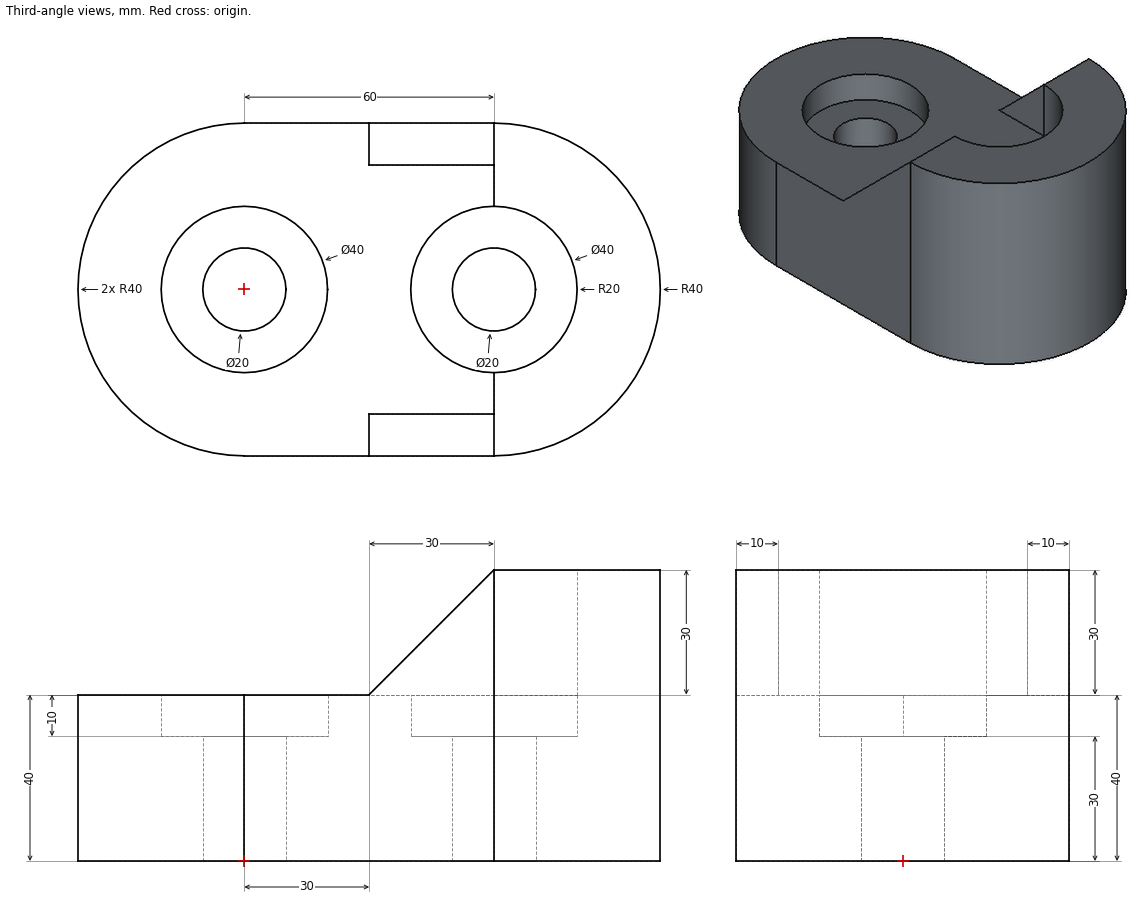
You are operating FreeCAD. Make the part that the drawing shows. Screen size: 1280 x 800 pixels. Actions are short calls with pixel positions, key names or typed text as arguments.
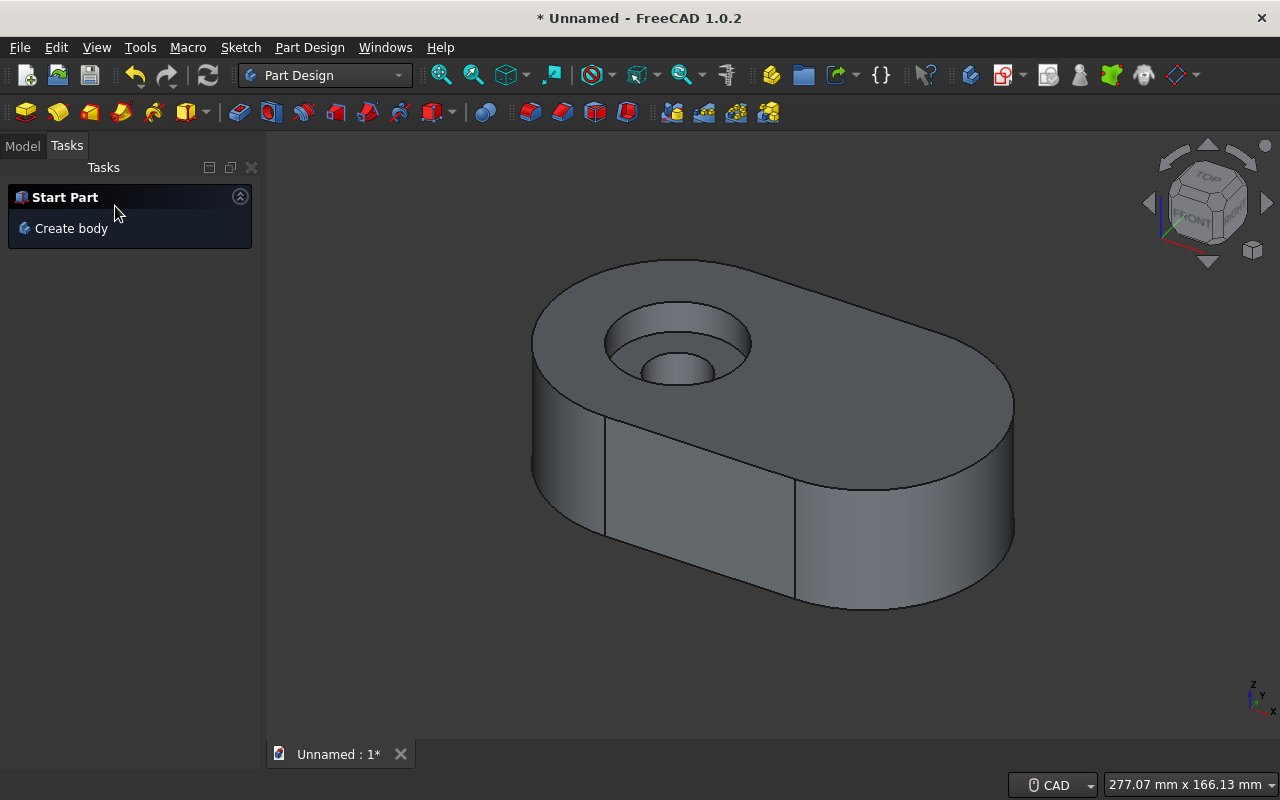
click(900, 416)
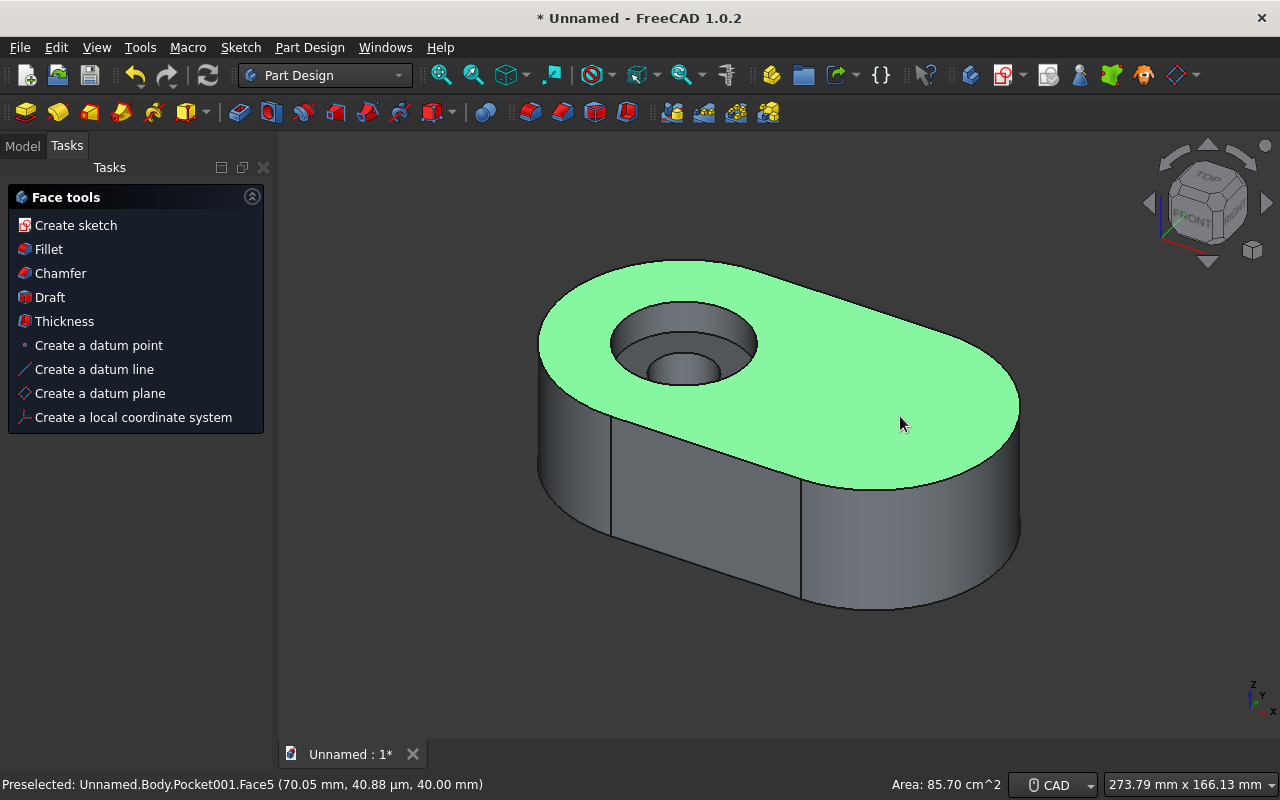
click(1004, 76)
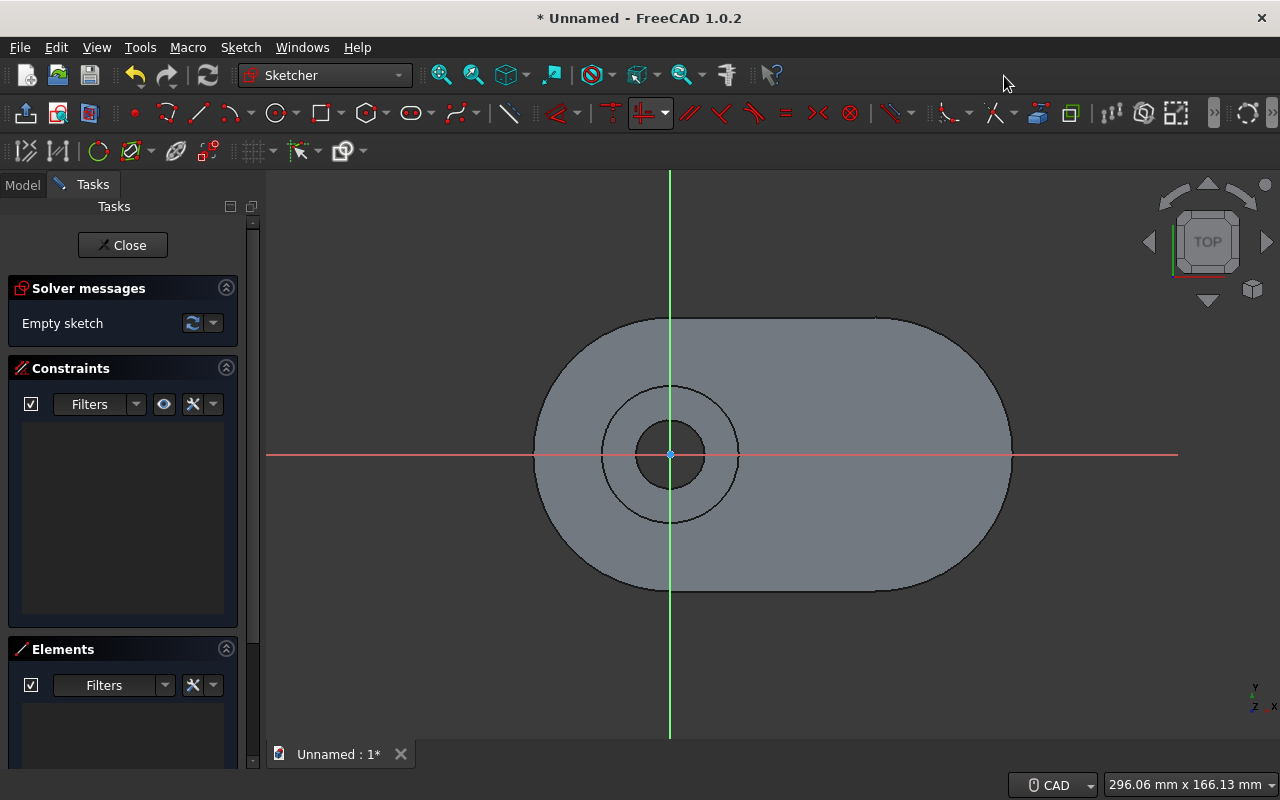
click(200, 114)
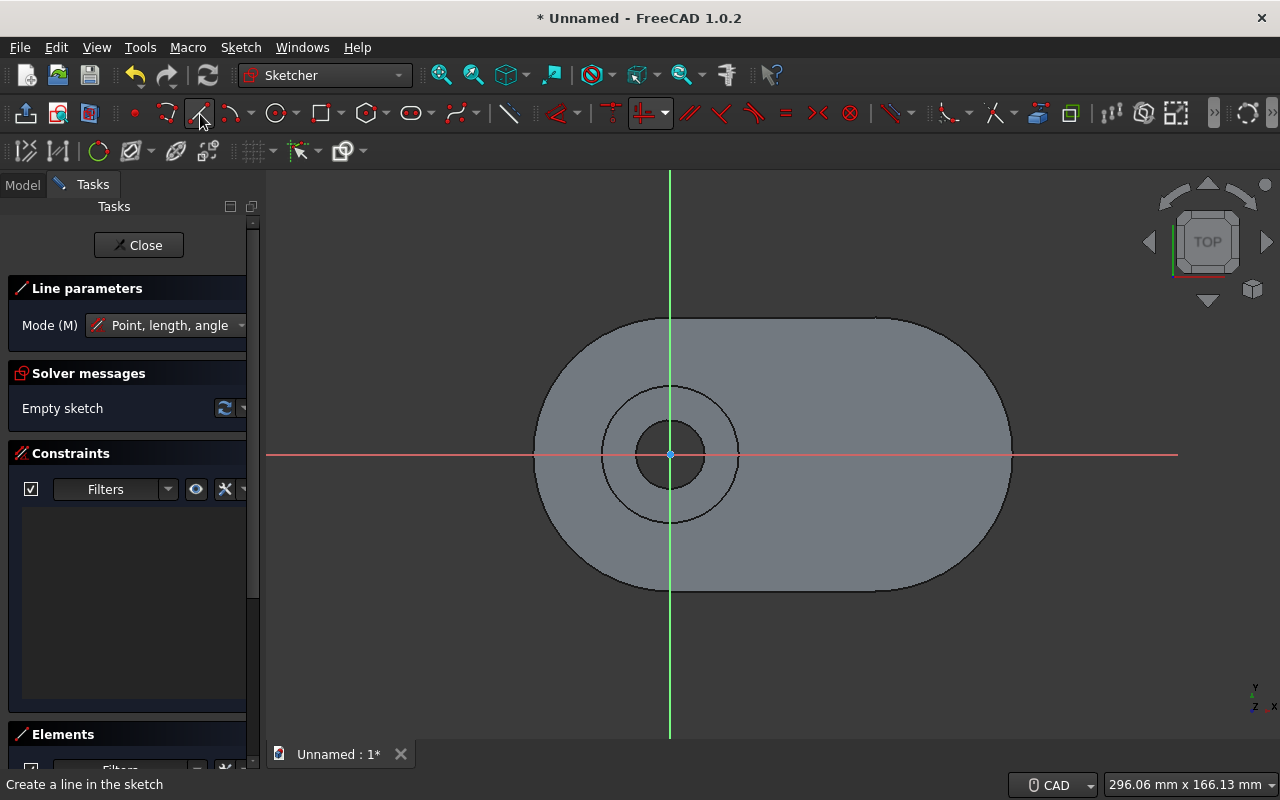
click(876, 318)
click(876, 591)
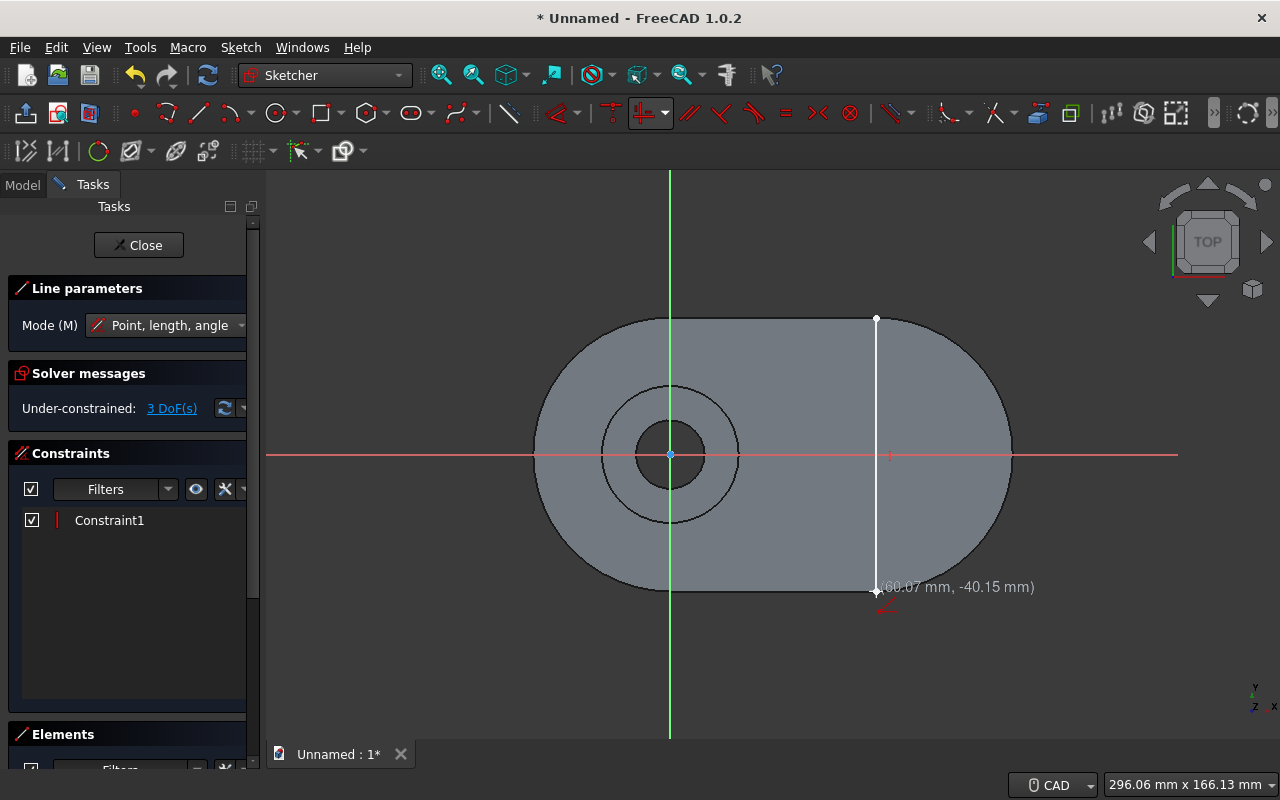
click(254, 114)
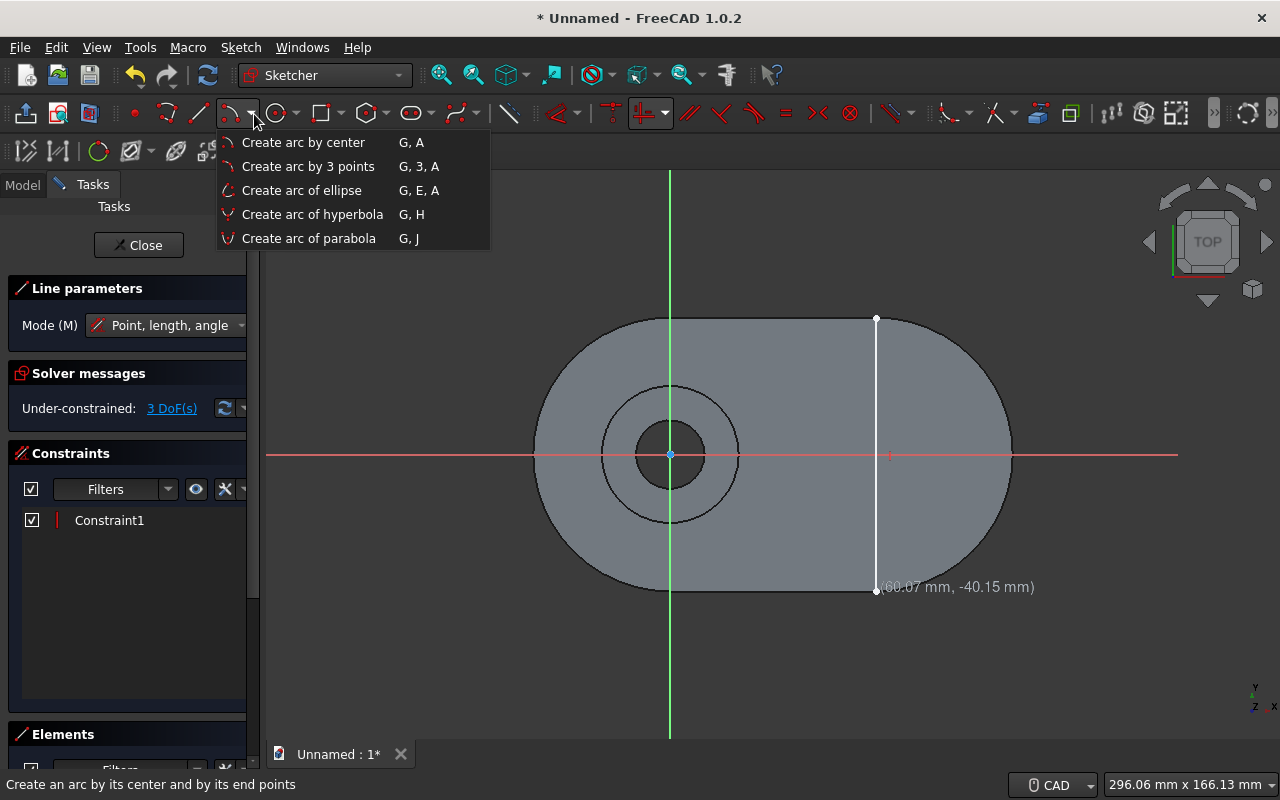
click(354, 166)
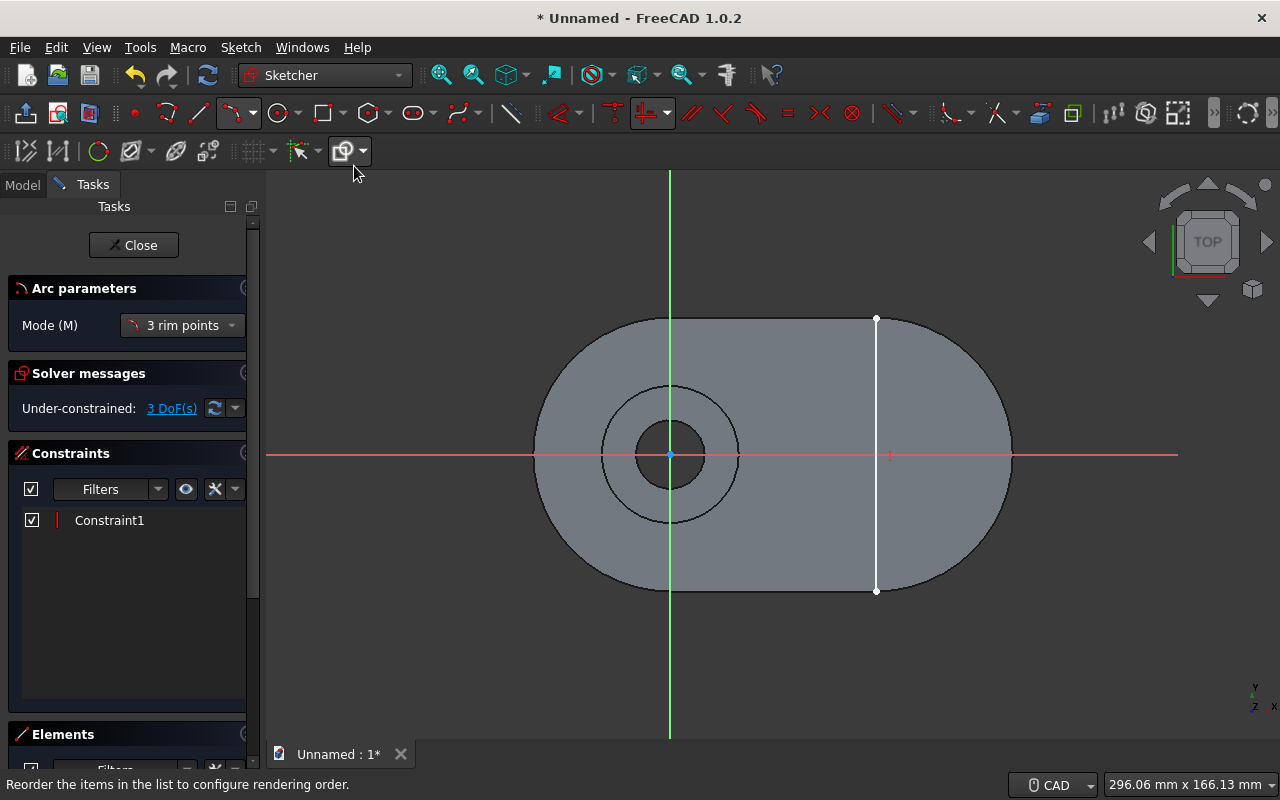
click(876, 592)
click(876, 319)
click(1006, 497)
key(Escape)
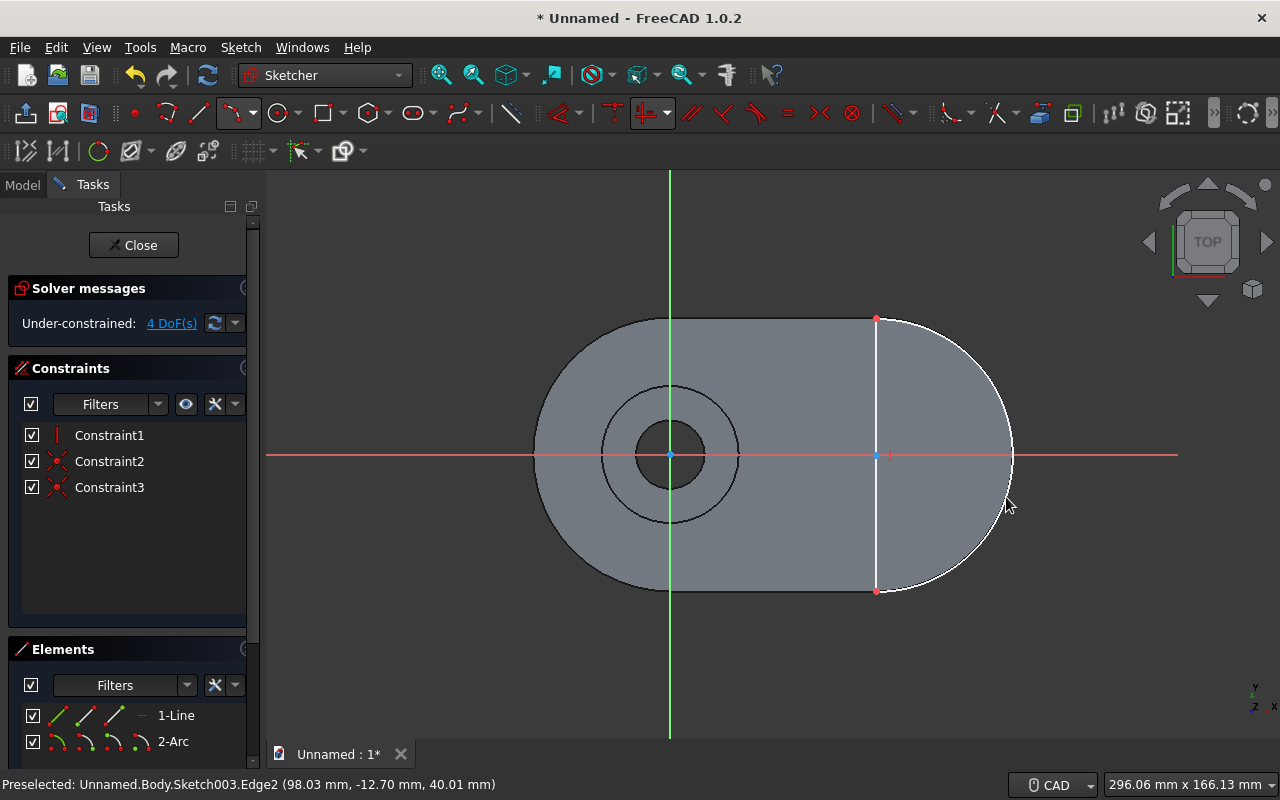
click(876, 455)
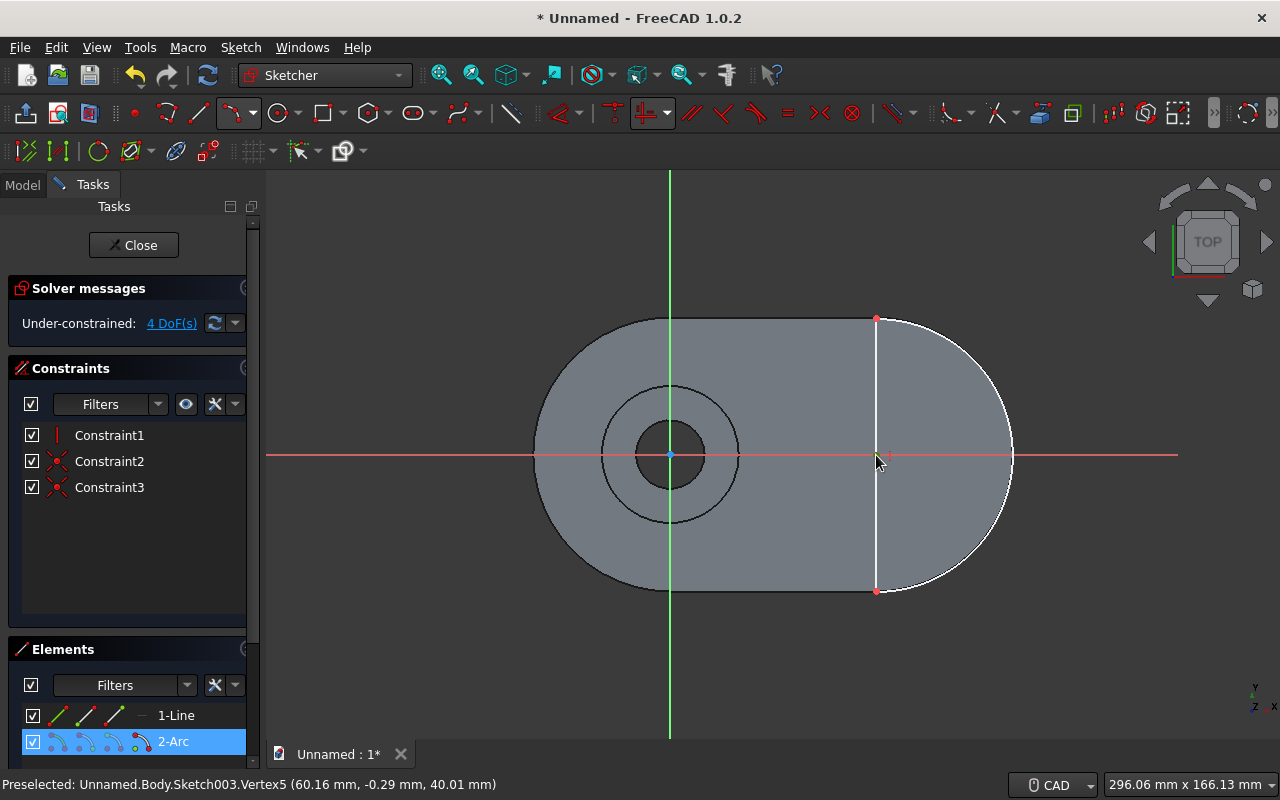
click(353, 455)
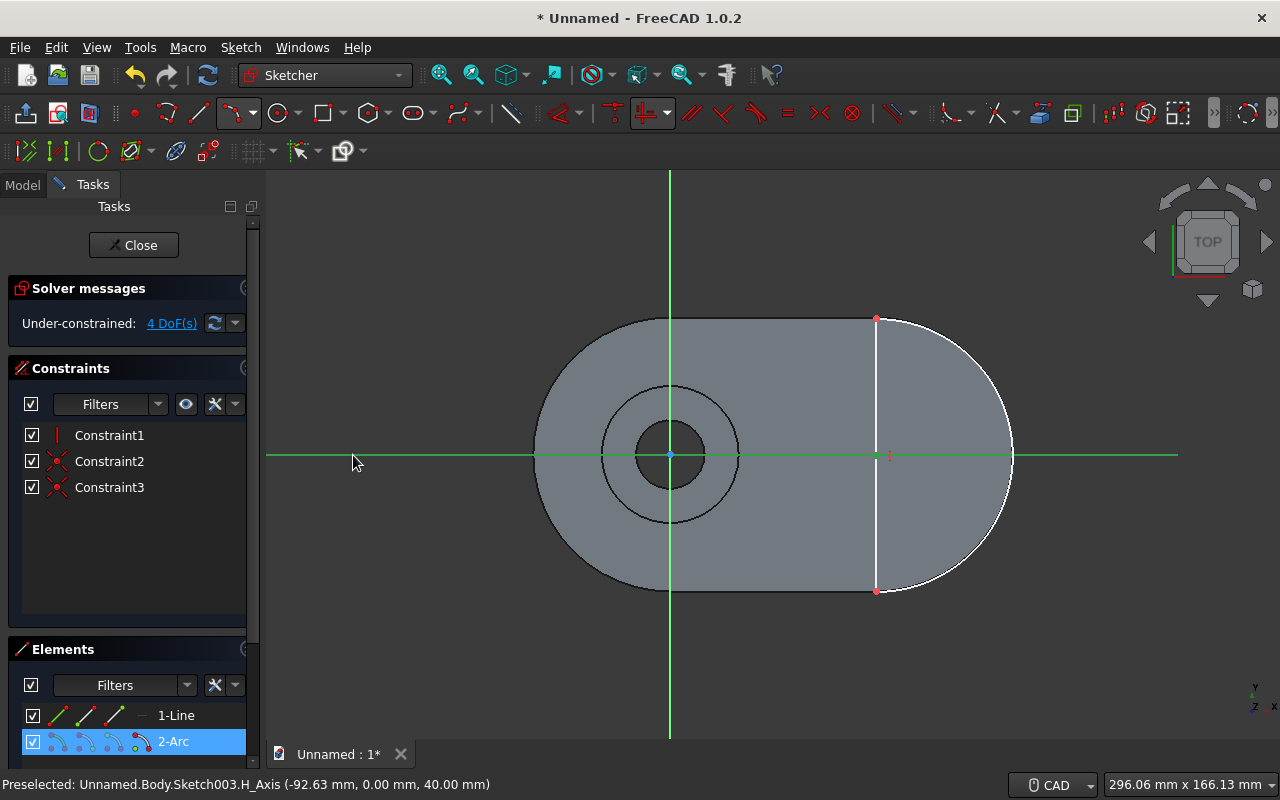
click(614, 114)